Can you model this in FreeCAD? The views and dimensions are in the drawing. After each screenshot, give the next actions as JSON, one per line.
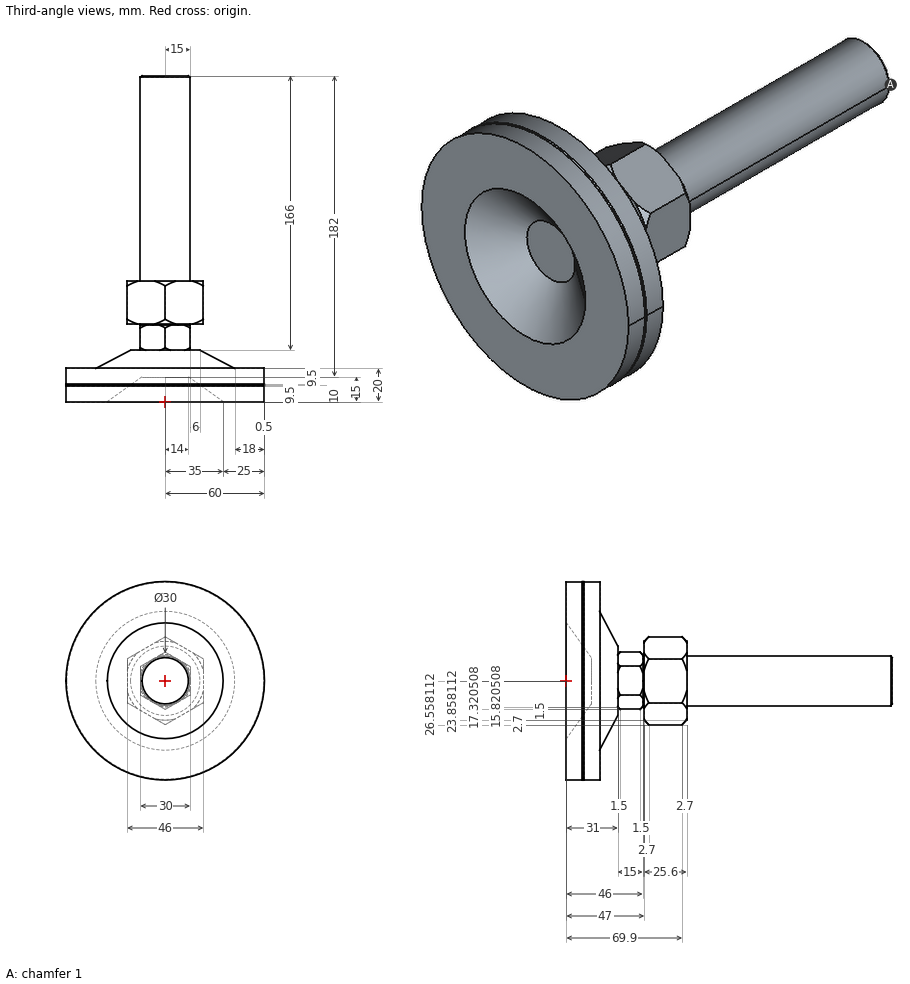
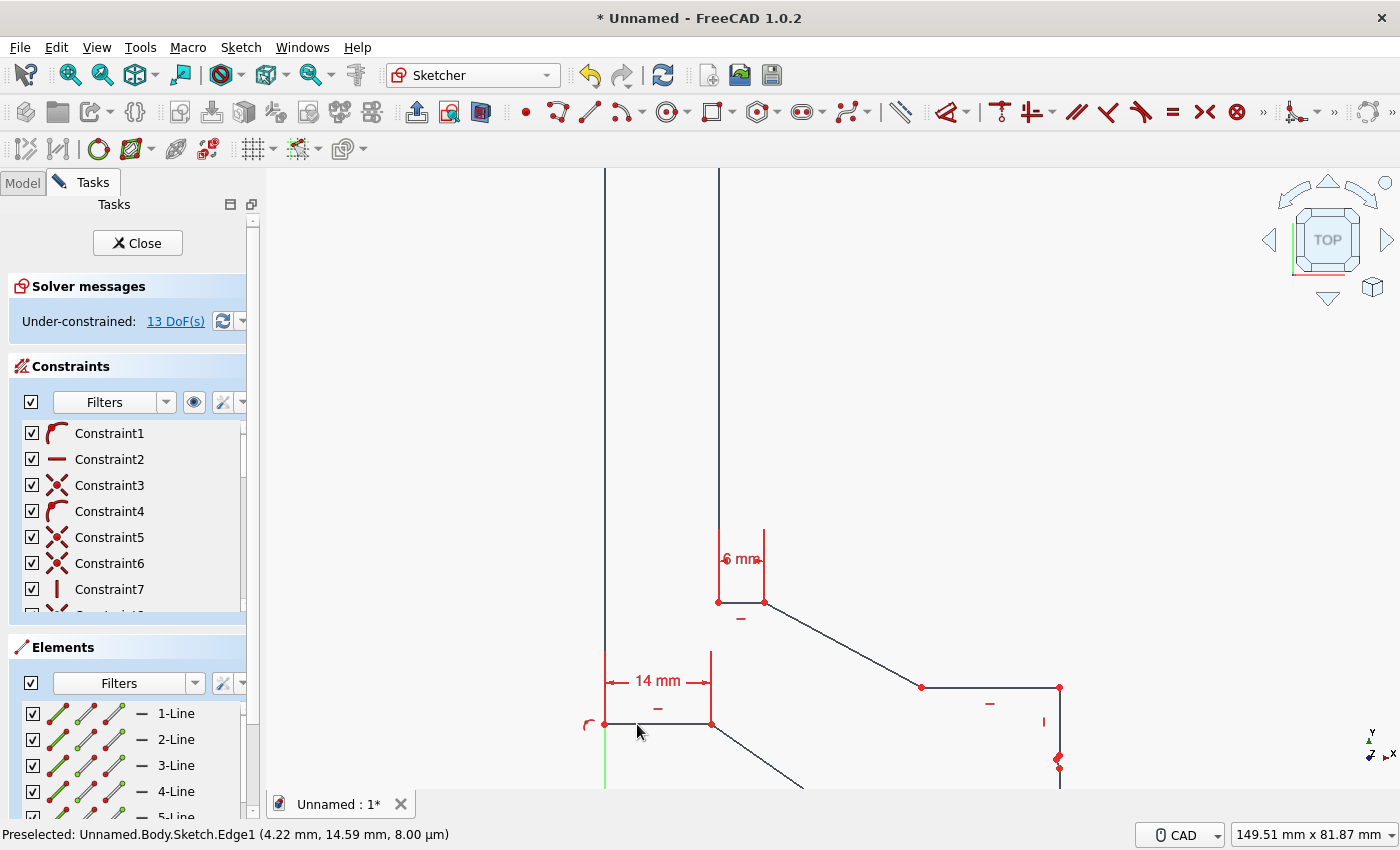
{"action": "scroll", "coordinate": [742, 606], "scroll_direction": "down", "scroll_amount": 7}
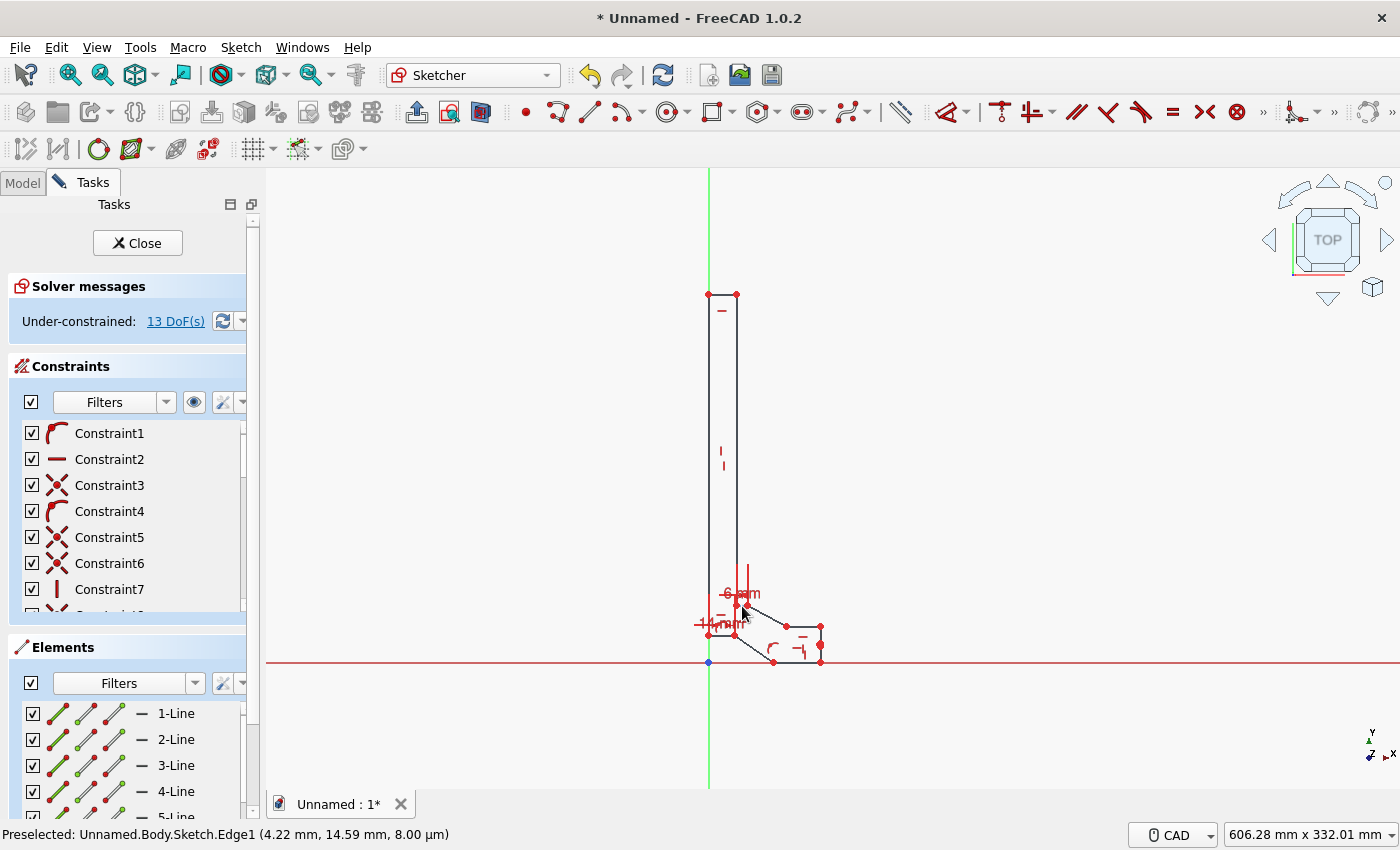
{"action": "left_click", "coordinate": [788, 663]}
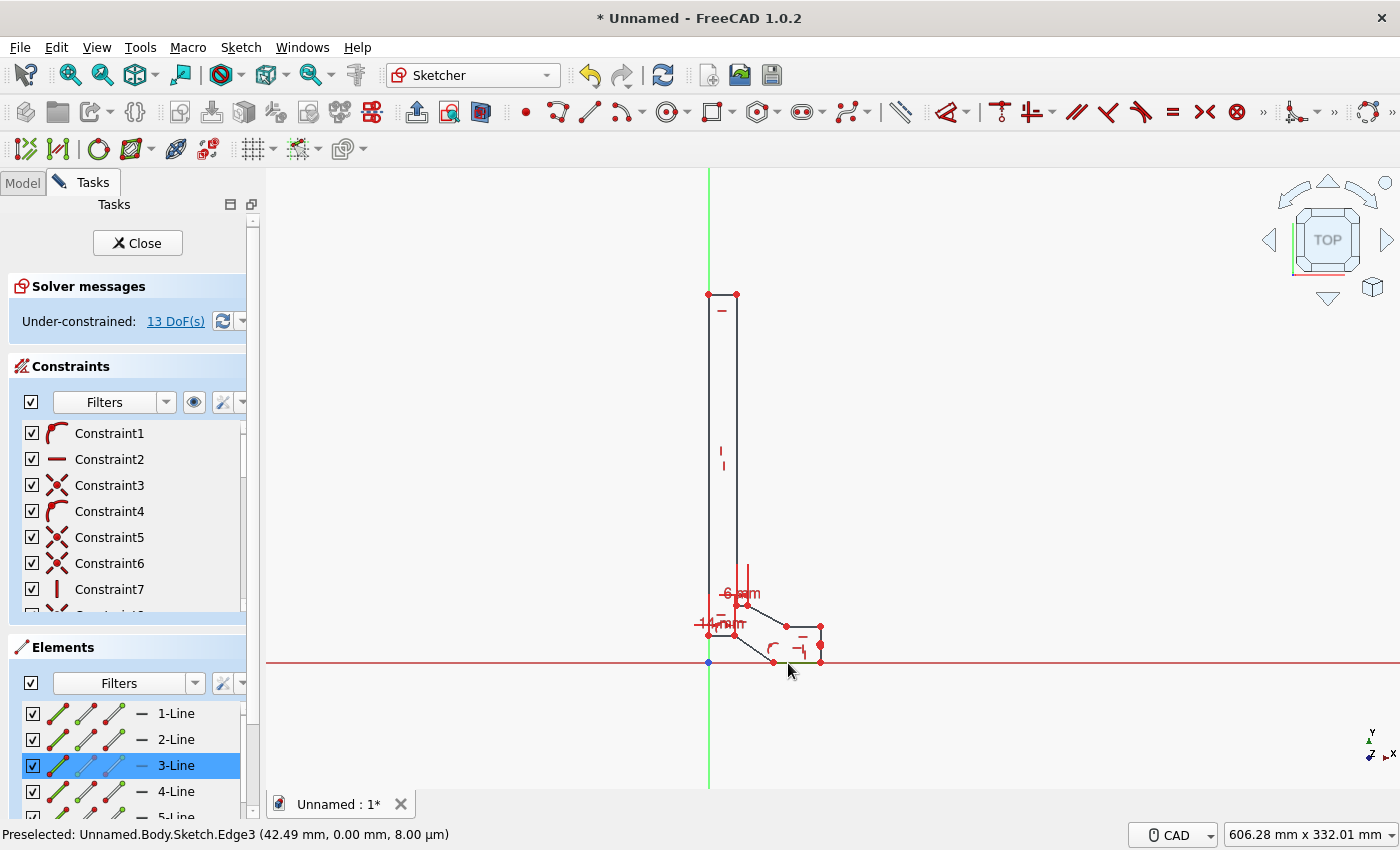
{"action": "key", "text": "l"}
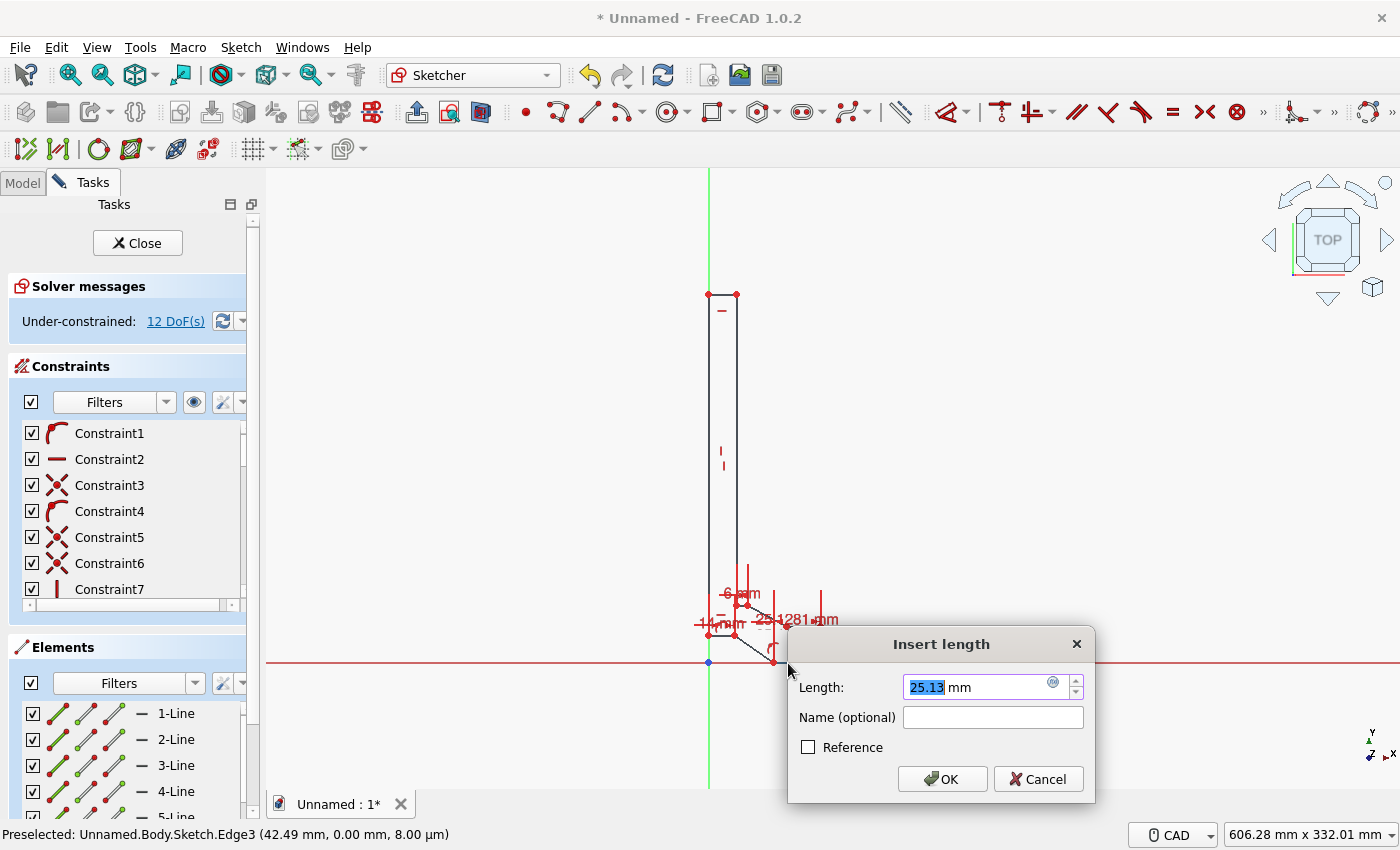
{"action": "type", "text": "25"}
{"action": "key", "text": "Return"}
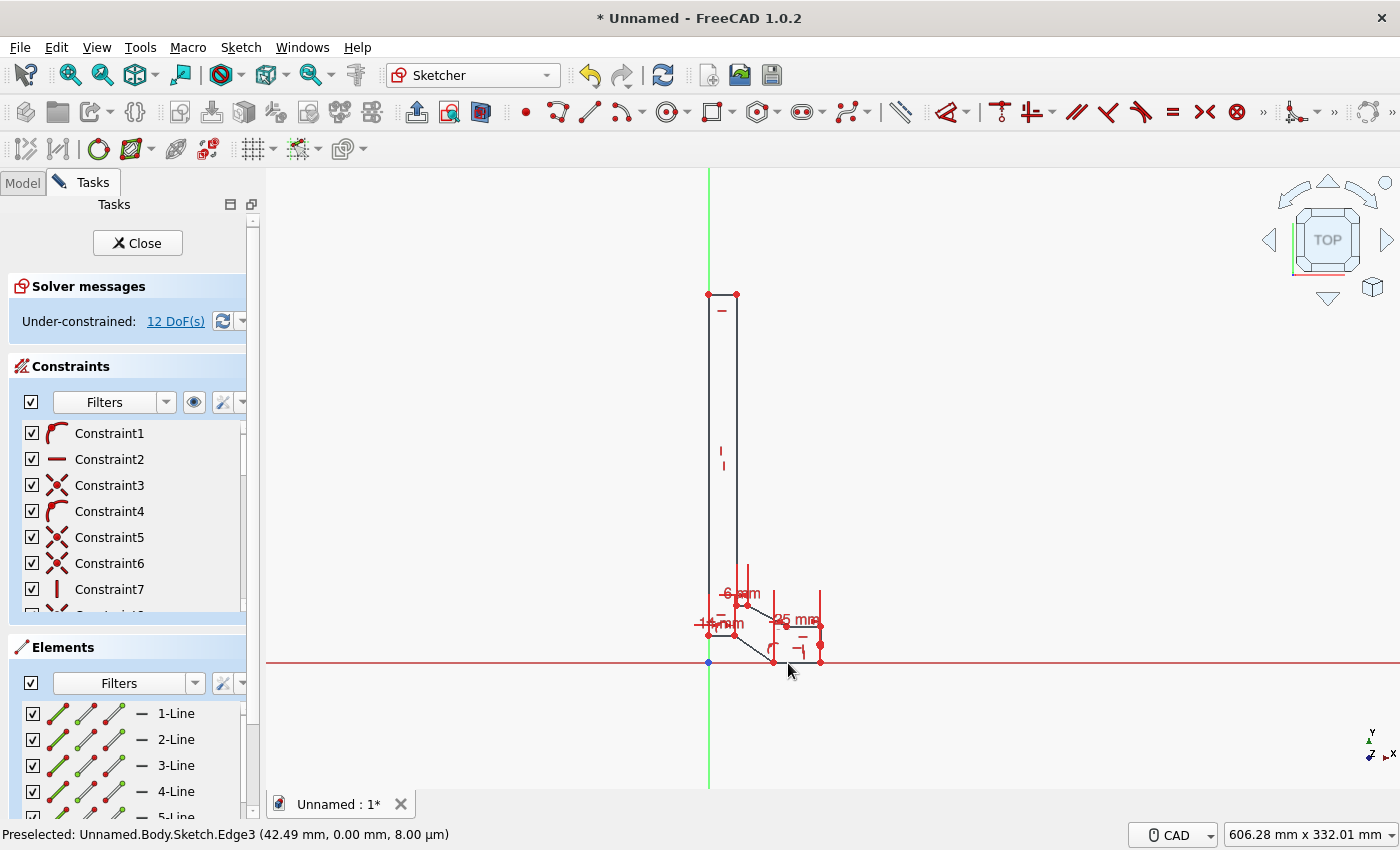
{"action": "scroll", "coordinate": [811, 627], "scroll_direction": "up", "scroll_amount": 2}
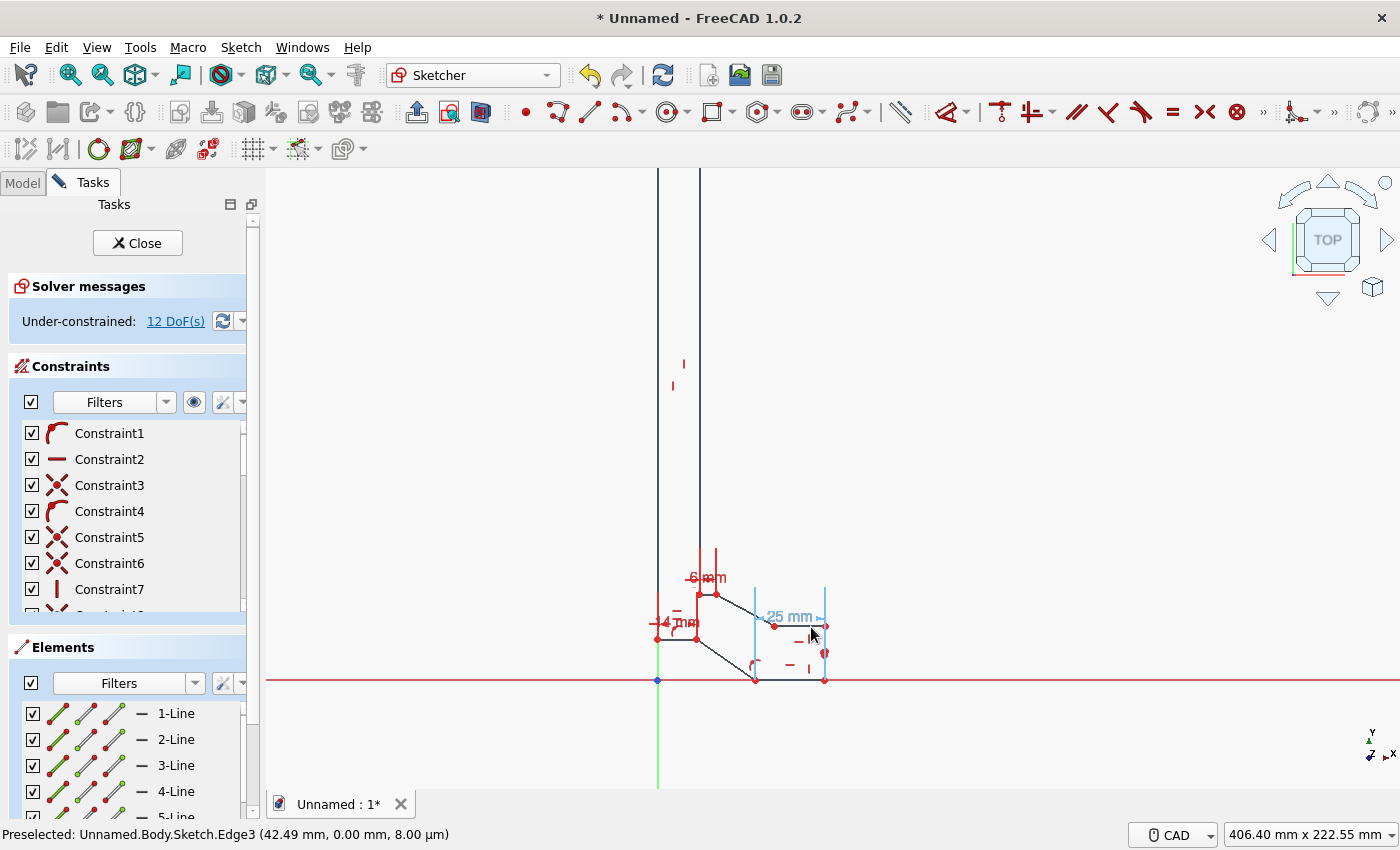
{"action": "left_click", "coordinate": [810, 626]}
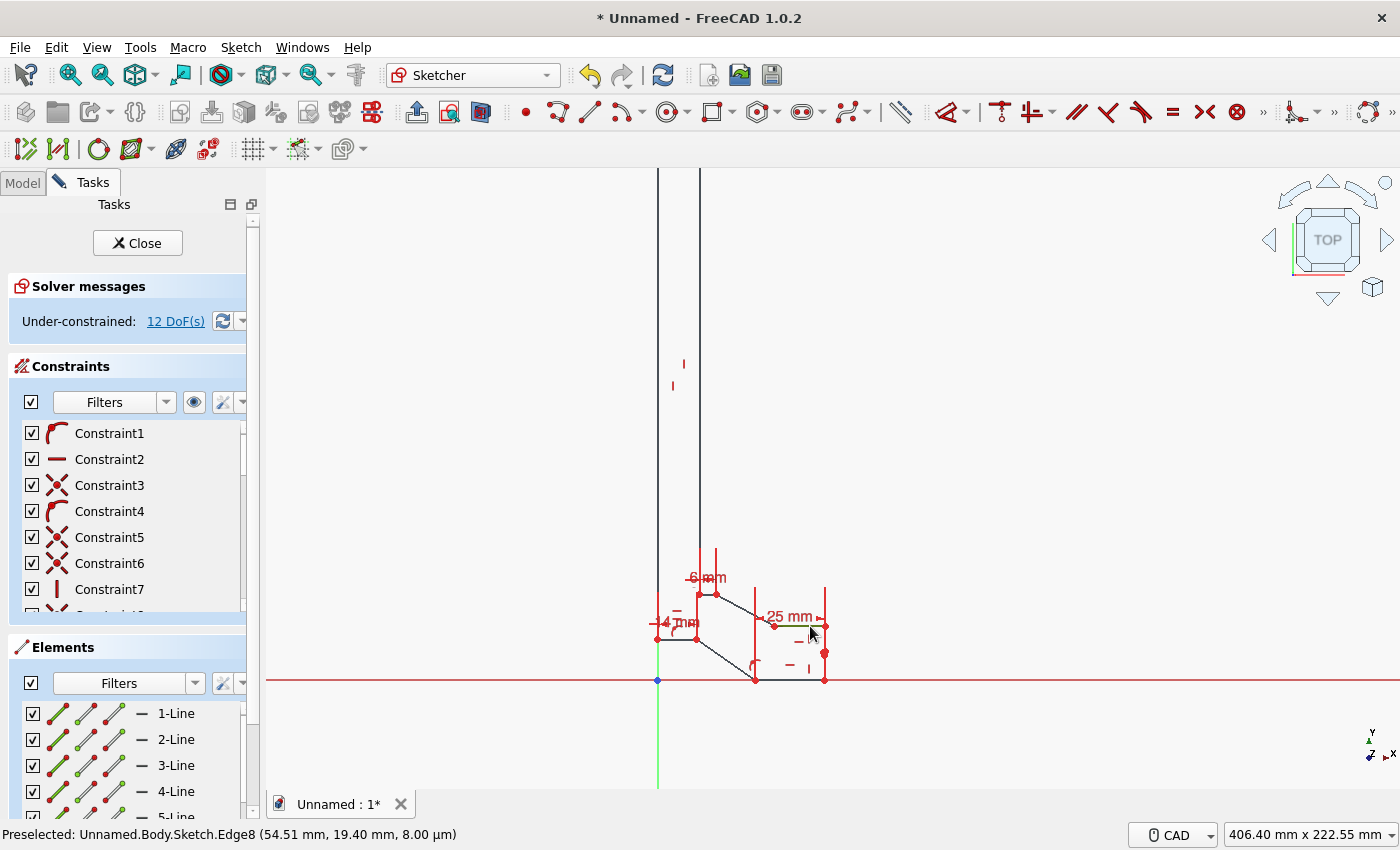
{"action": "key", "text": "l"}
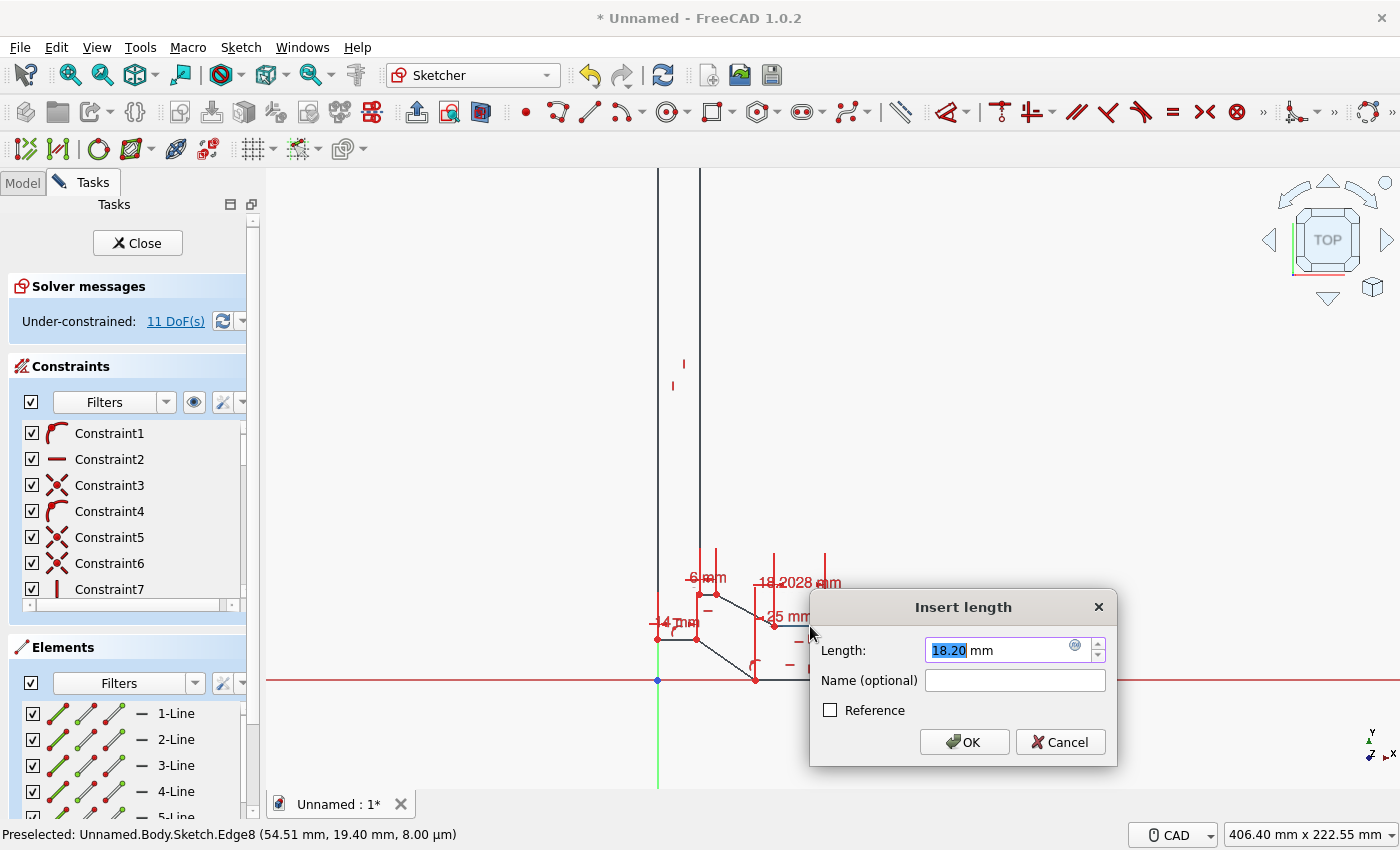
{"action": "type", "text": "18"}
{"action": "key", "text": "Return"}